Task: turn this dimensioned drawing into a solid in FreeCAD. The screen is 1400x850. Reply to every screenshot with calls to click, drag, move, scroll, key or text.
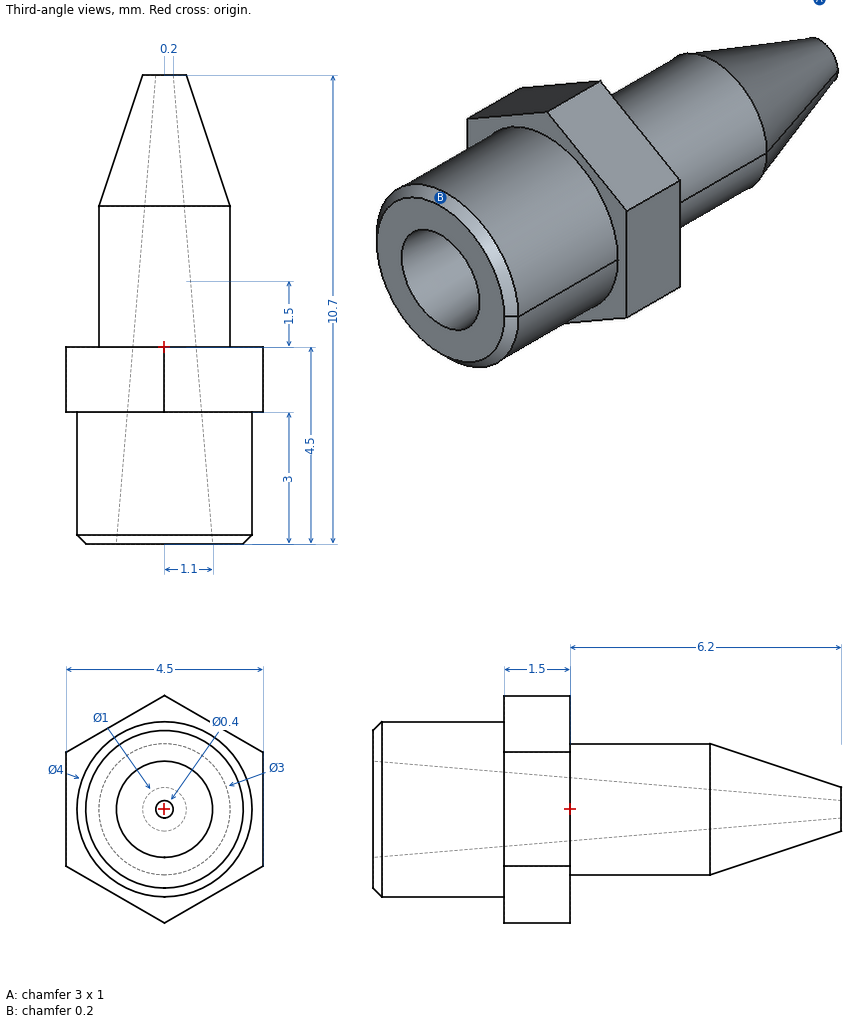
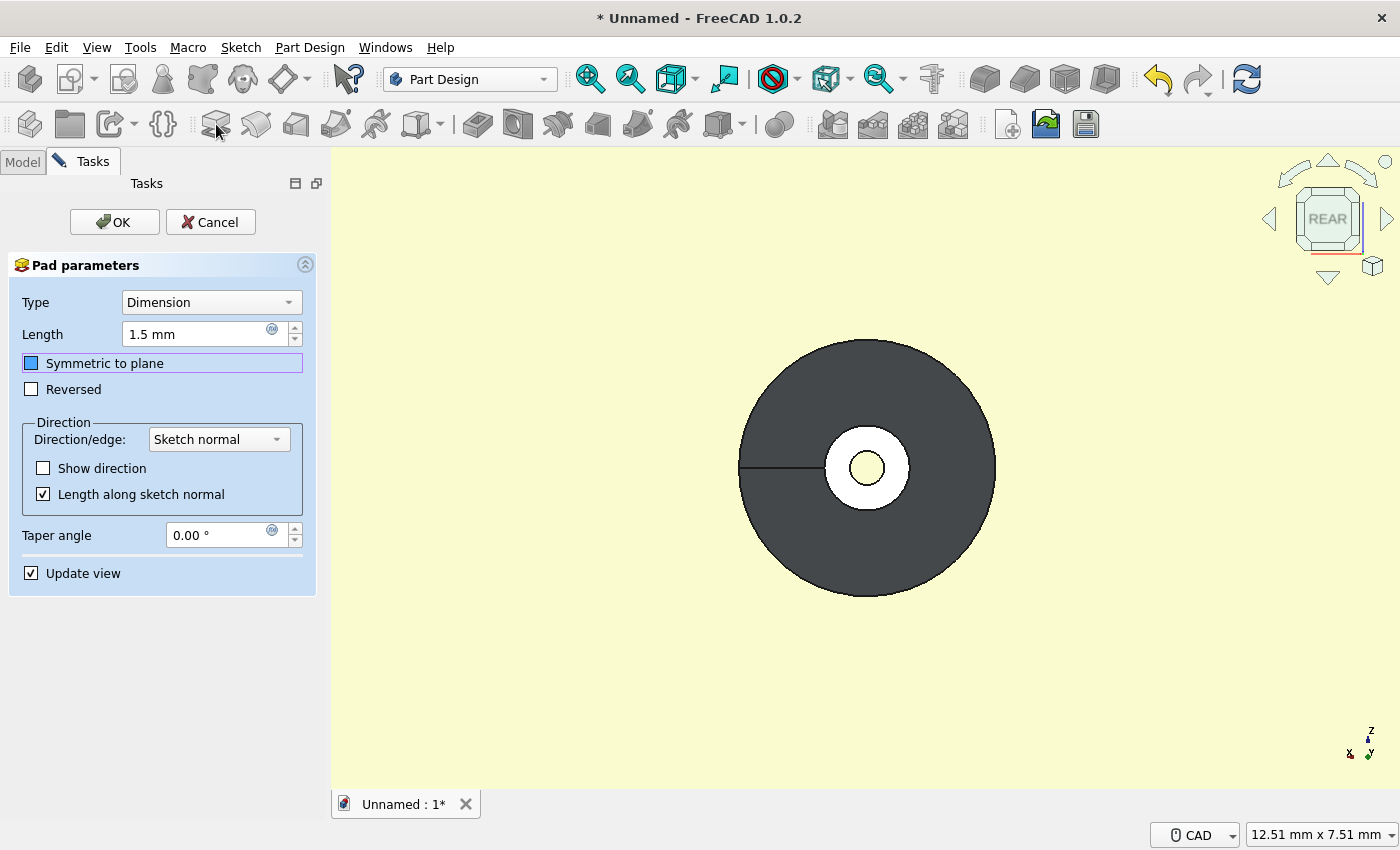
click(30, 389)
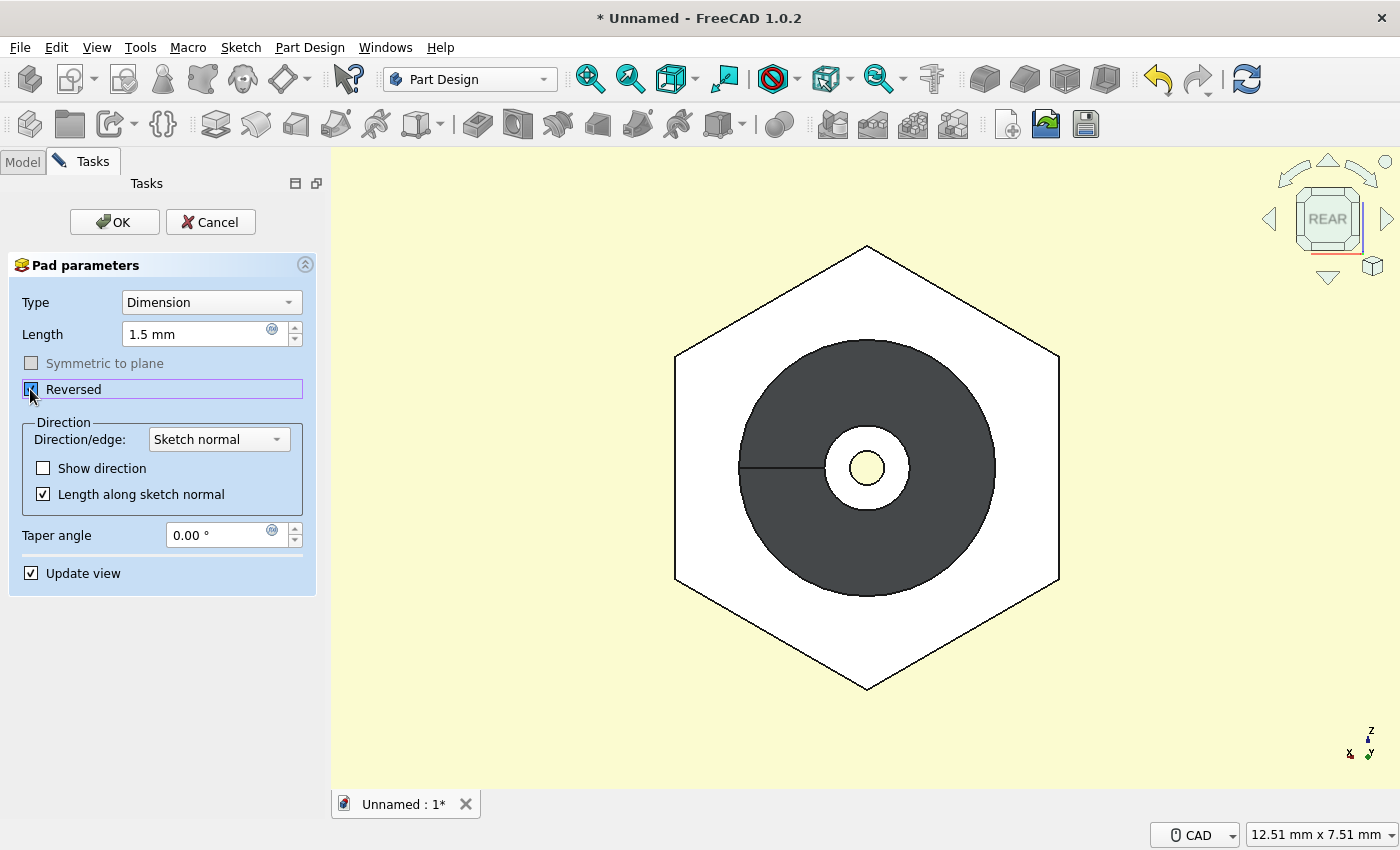
click(115, 222)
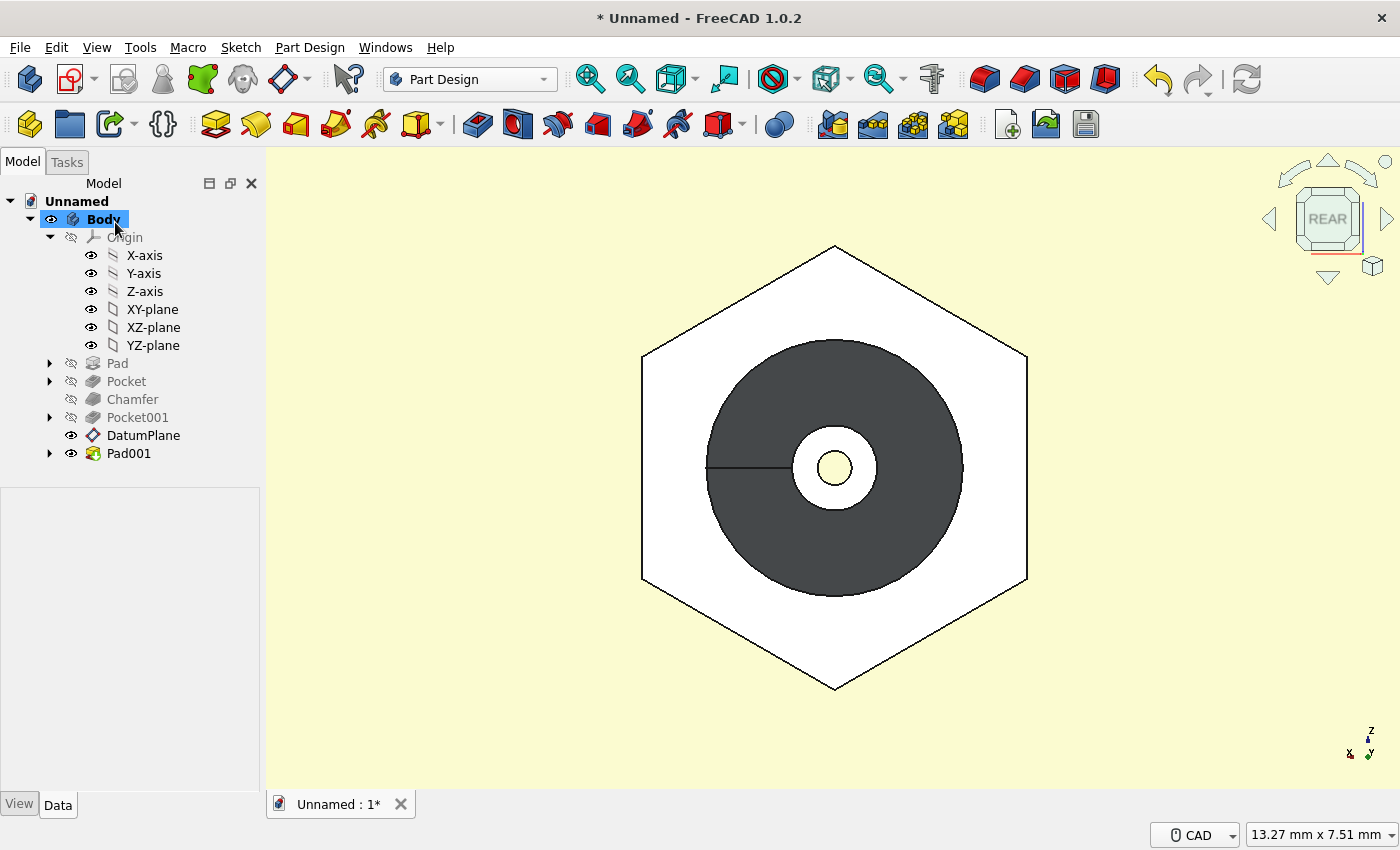
click(116, 435)
key(space)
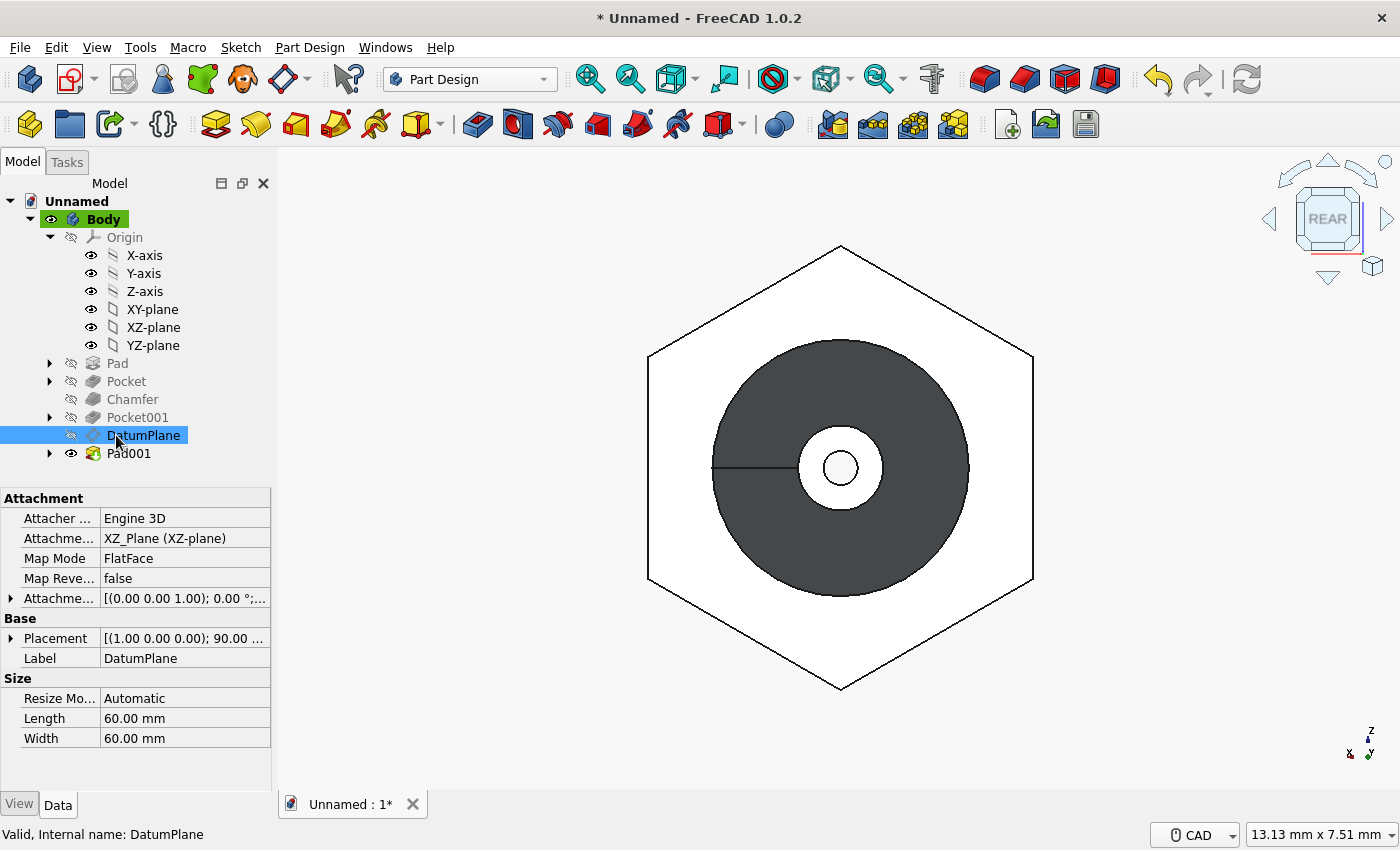
click(136, 327)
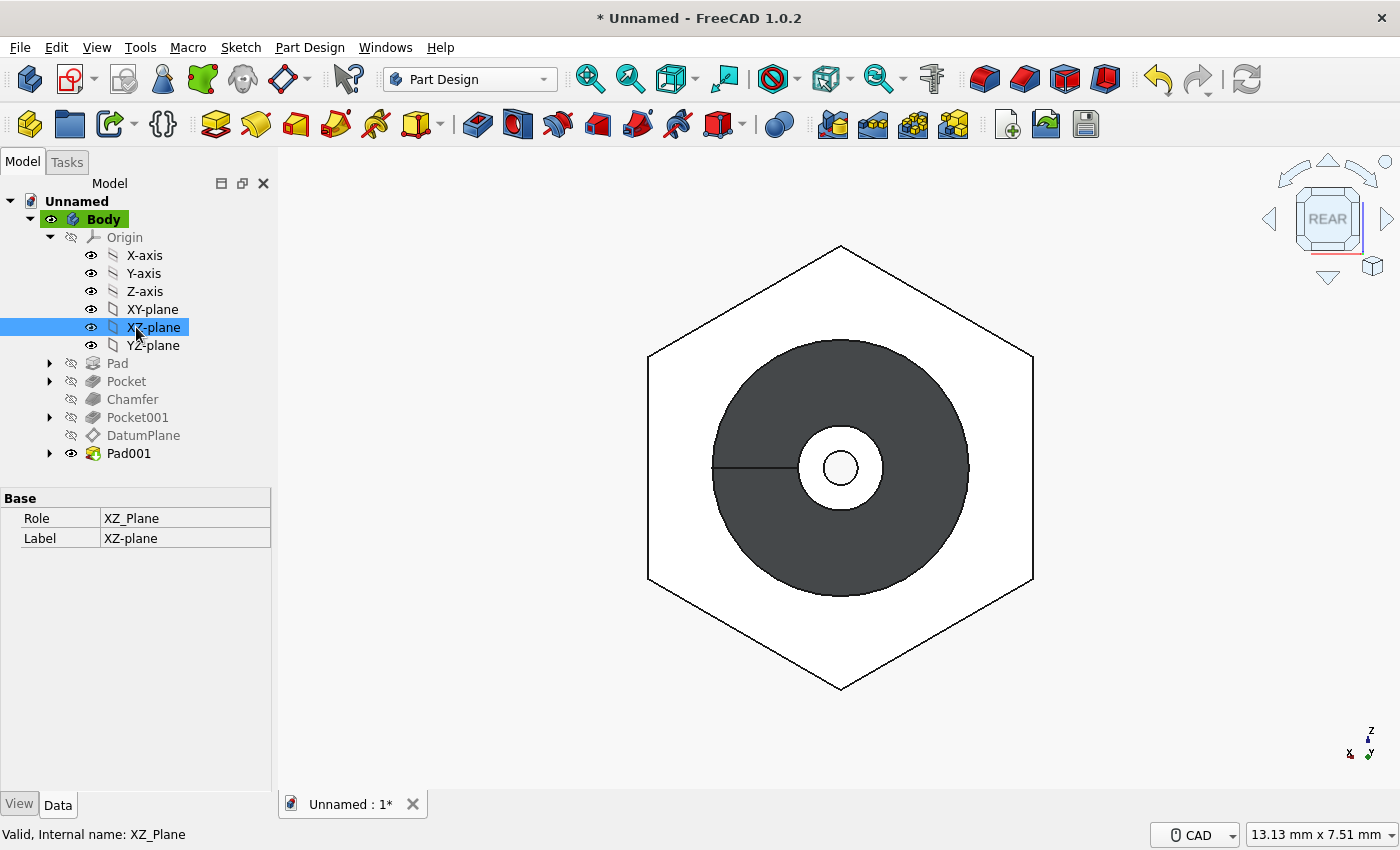
click(284, 80)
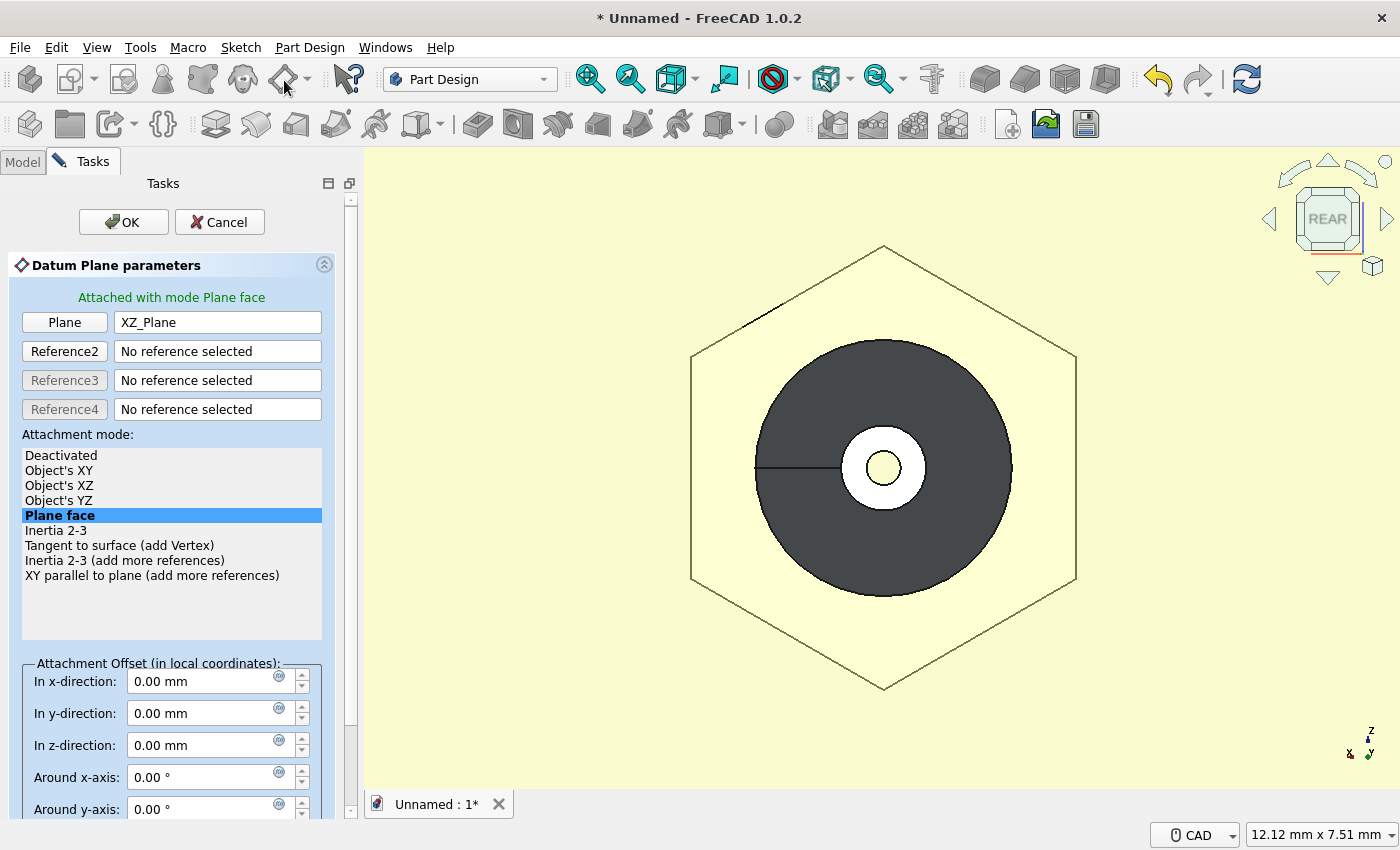
triple_click(210, 745)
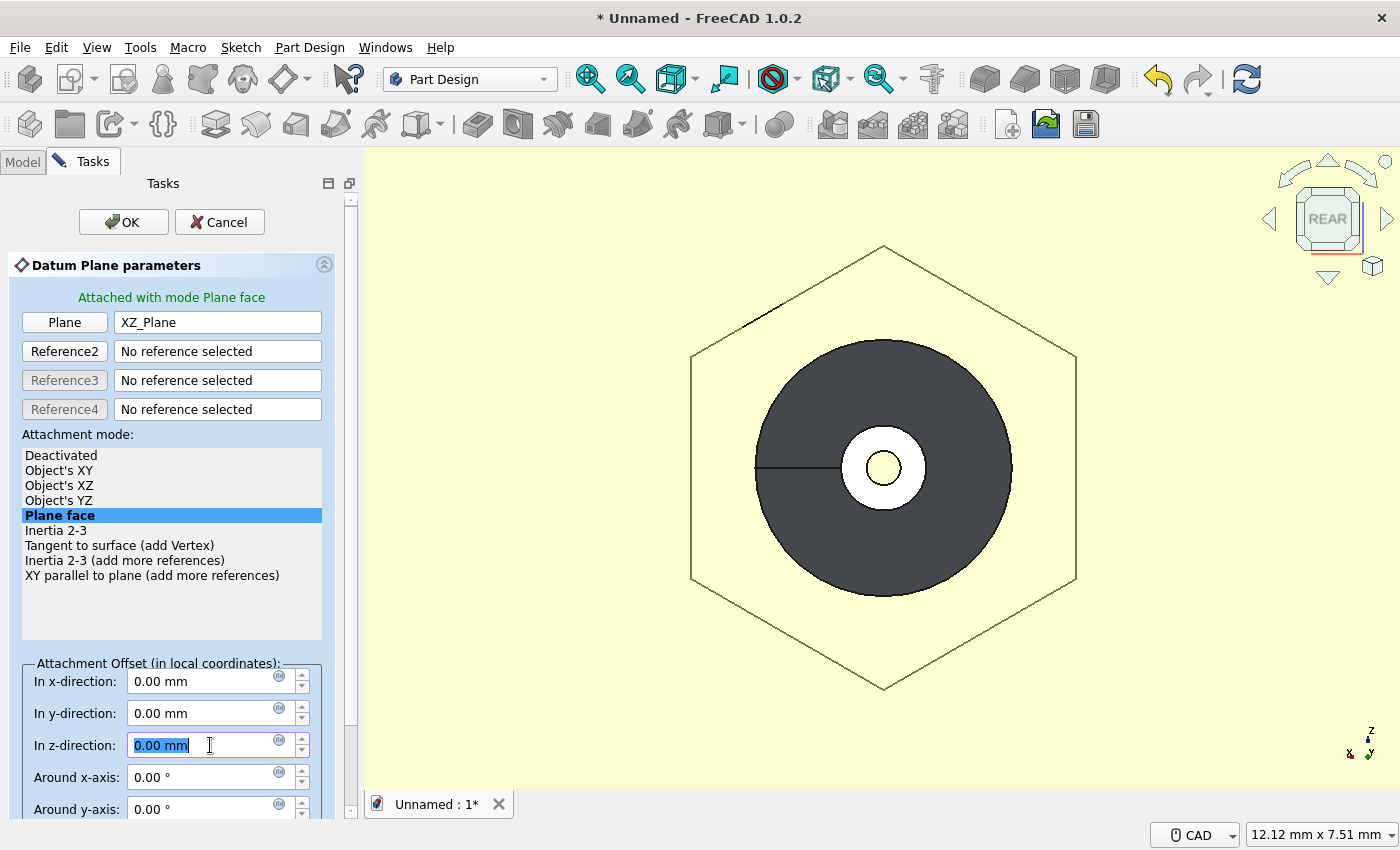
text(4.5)
key(Tab)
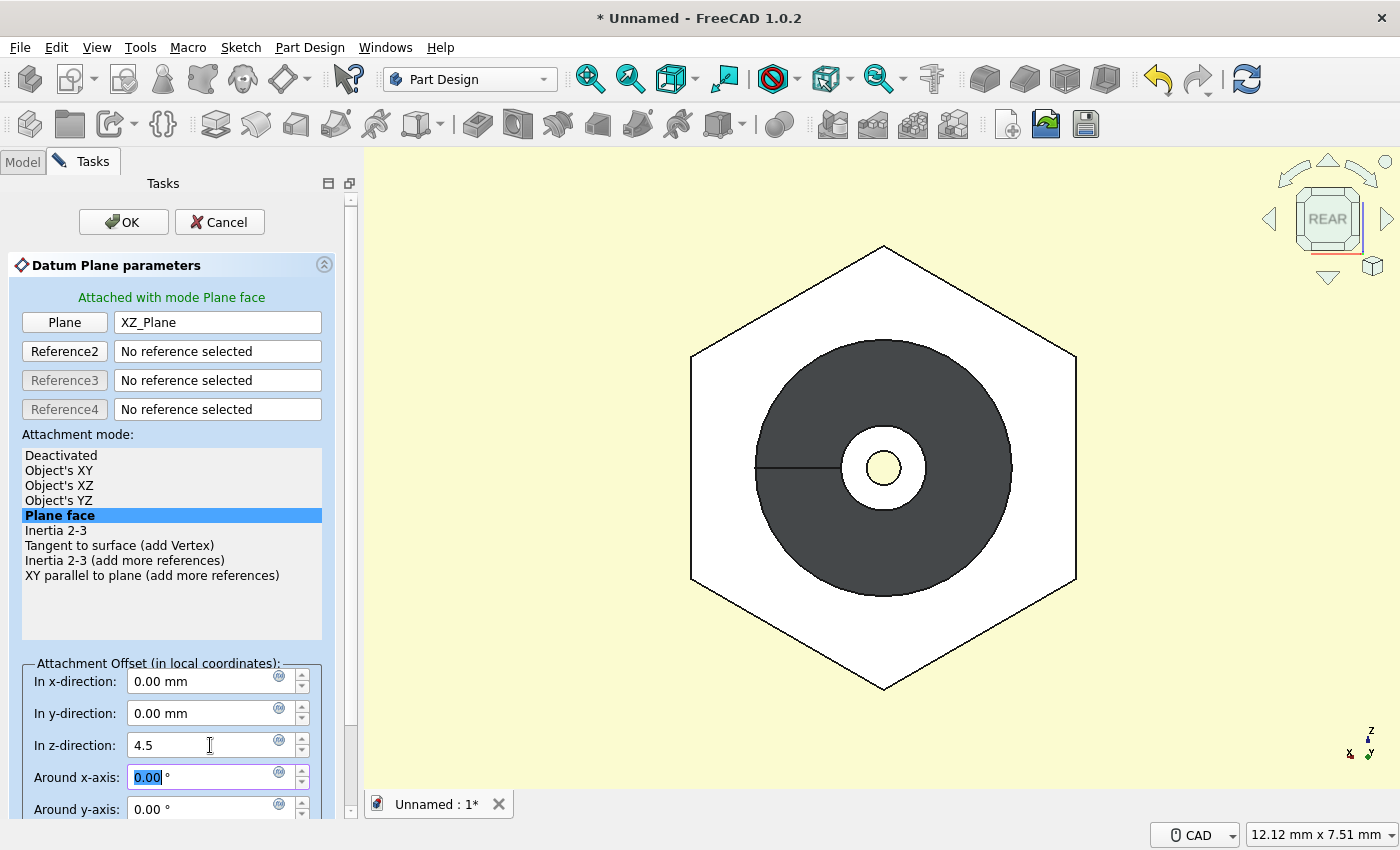
click(124, 222)